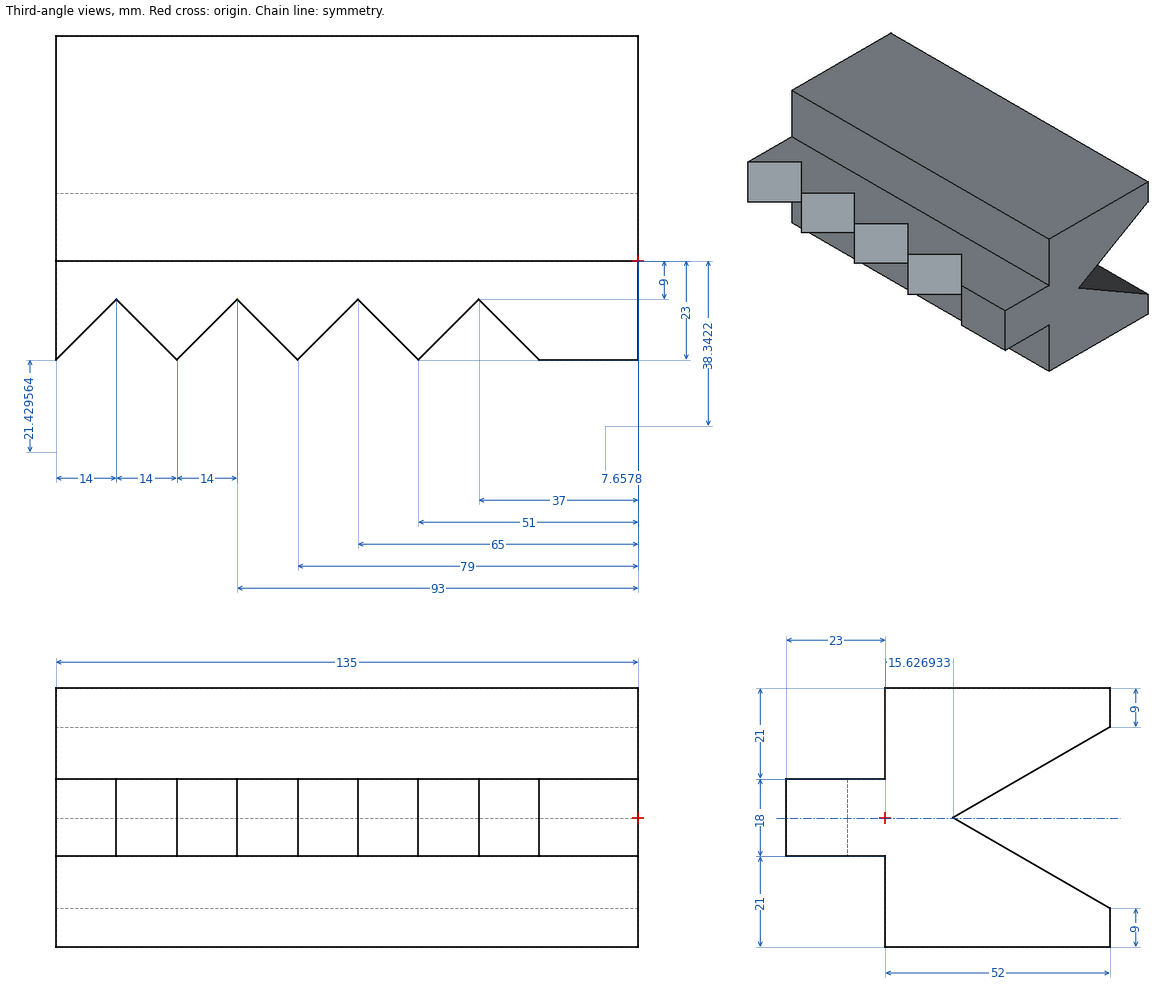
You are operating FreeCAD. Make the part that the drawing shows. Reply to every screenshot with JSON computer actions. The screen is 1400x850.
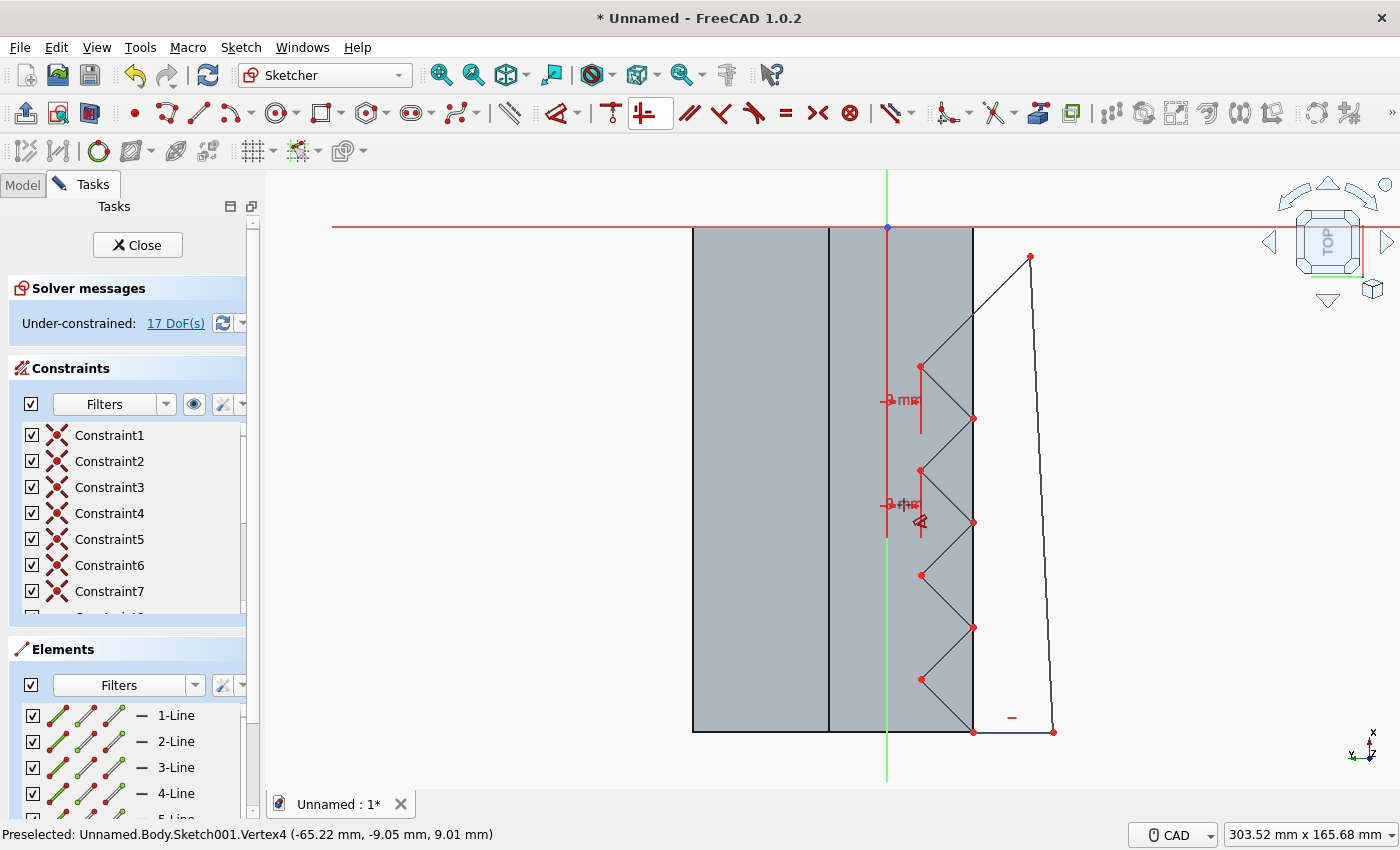
{"action": "left_click", "coordinate": [921, 576]}
{"action": "left_click", "coordinate": [904, 610]}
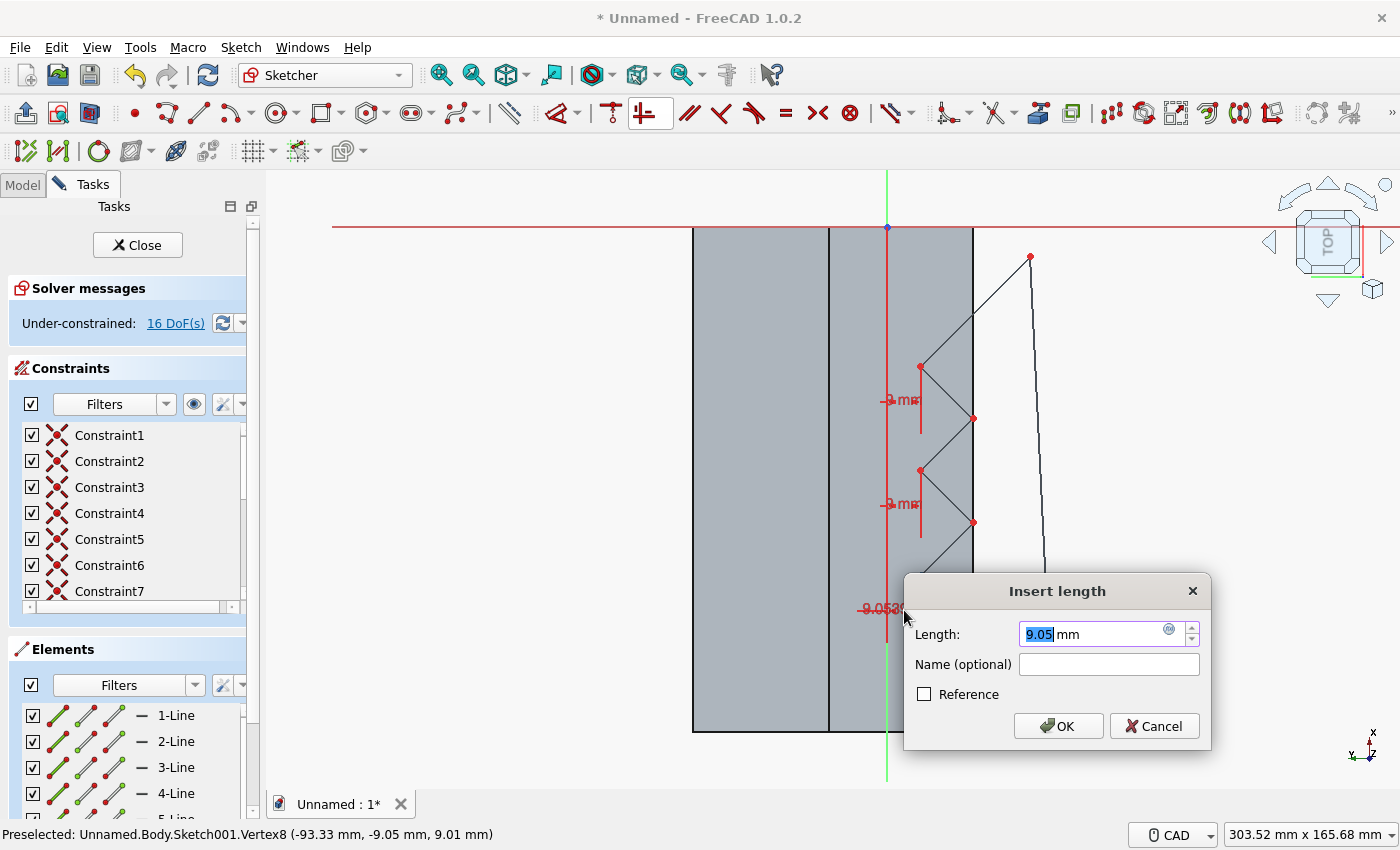
{"action": "type", "text": "9"}
{"action": "key", "text": "Return"}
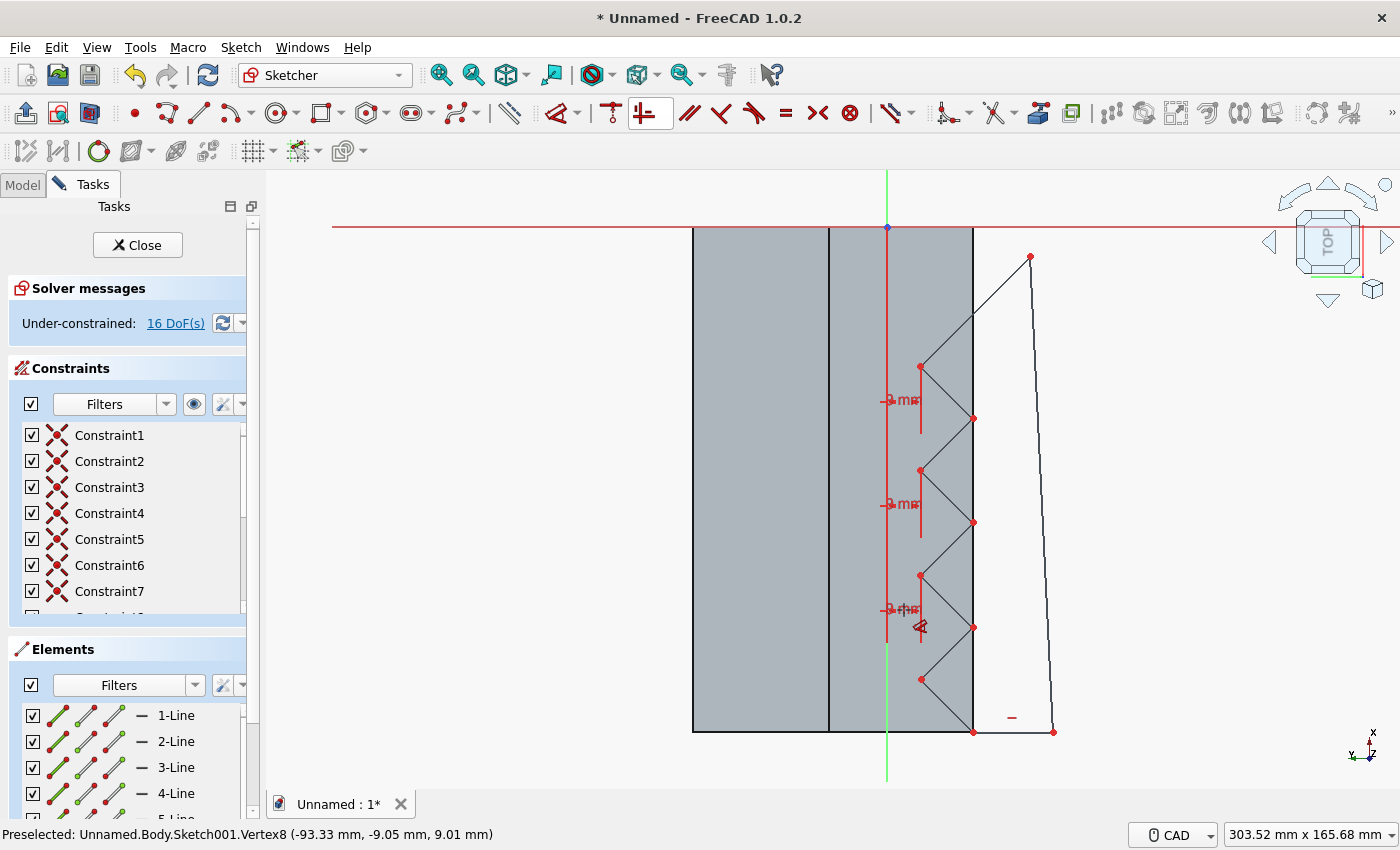
{"action": "left_click", "coordinate": [921, 680]}
{"action": "left_click", "coordinate": [904, 714]}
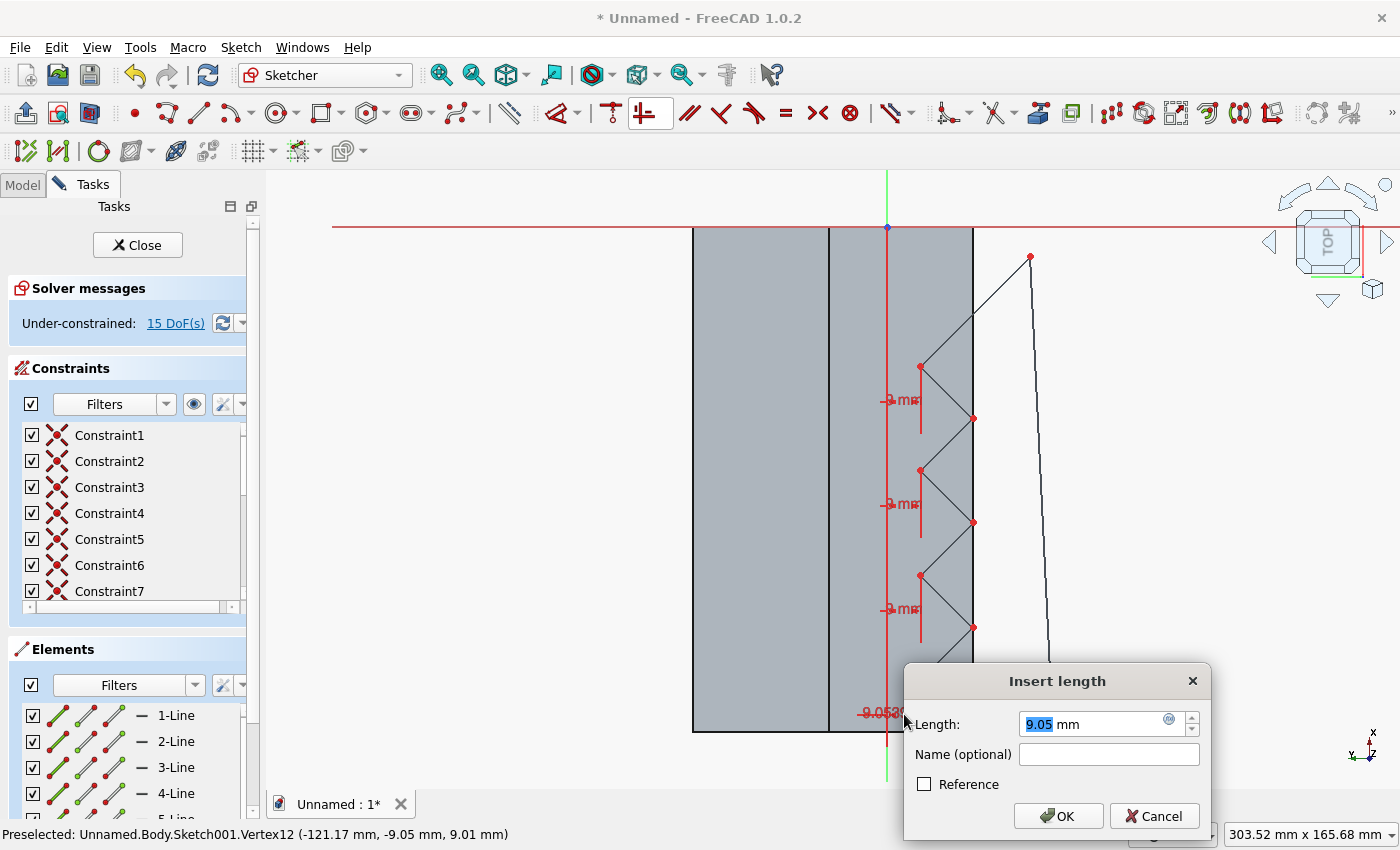
{"action": "type", "text": "9"}
{"action": "key", "text": "Return"}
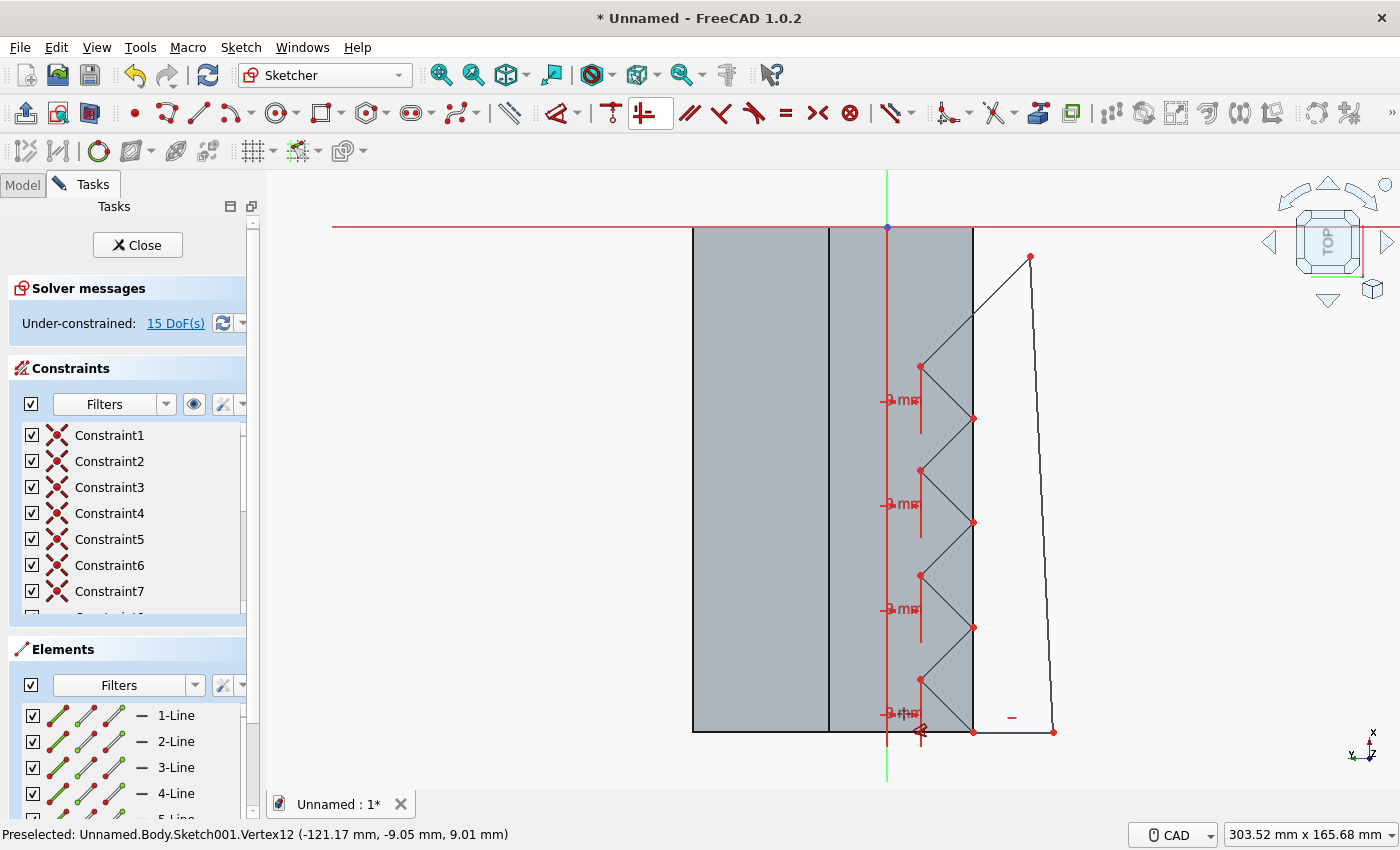
{"action": "left_click", "coordinate": [921, 367]}
{"action": "left_click", "coordinate": [853, 297]}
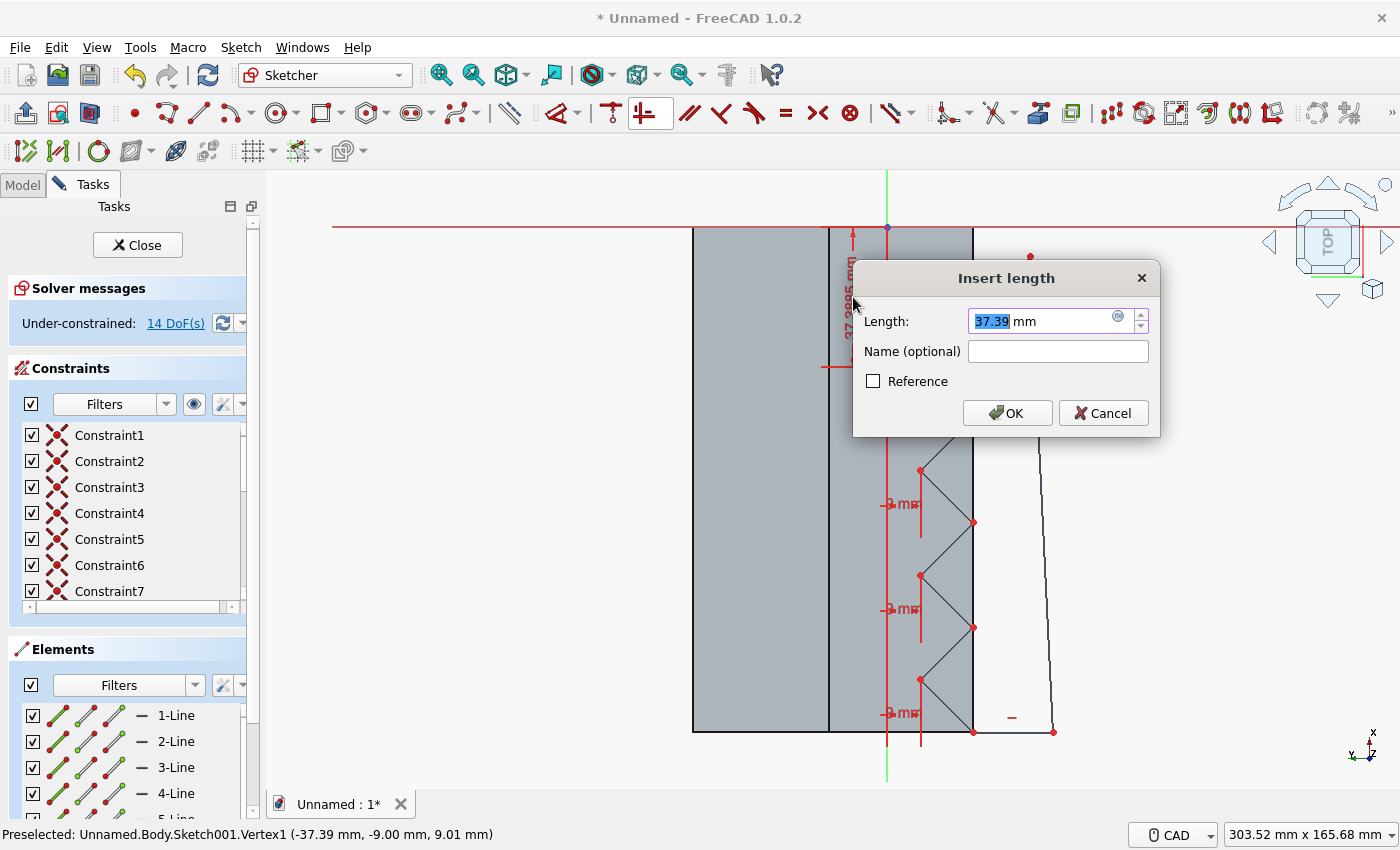
{"action": "type", "text": "37"}
{"action": "key", "text": "Return"}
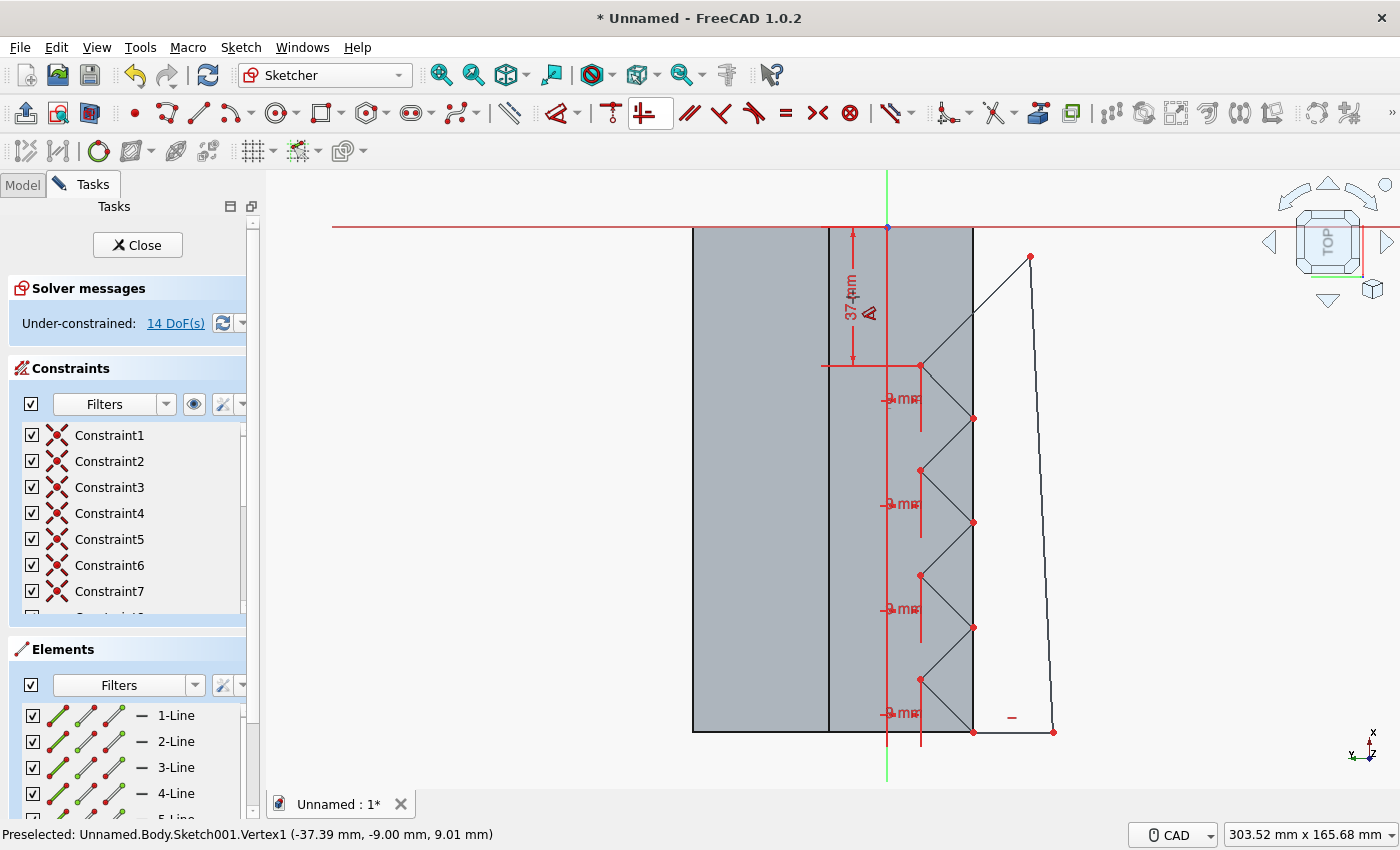
{"action": "left_click", "coordinate": [973, 419]}
{"action": "left_click", "coordinate": [910, 453]}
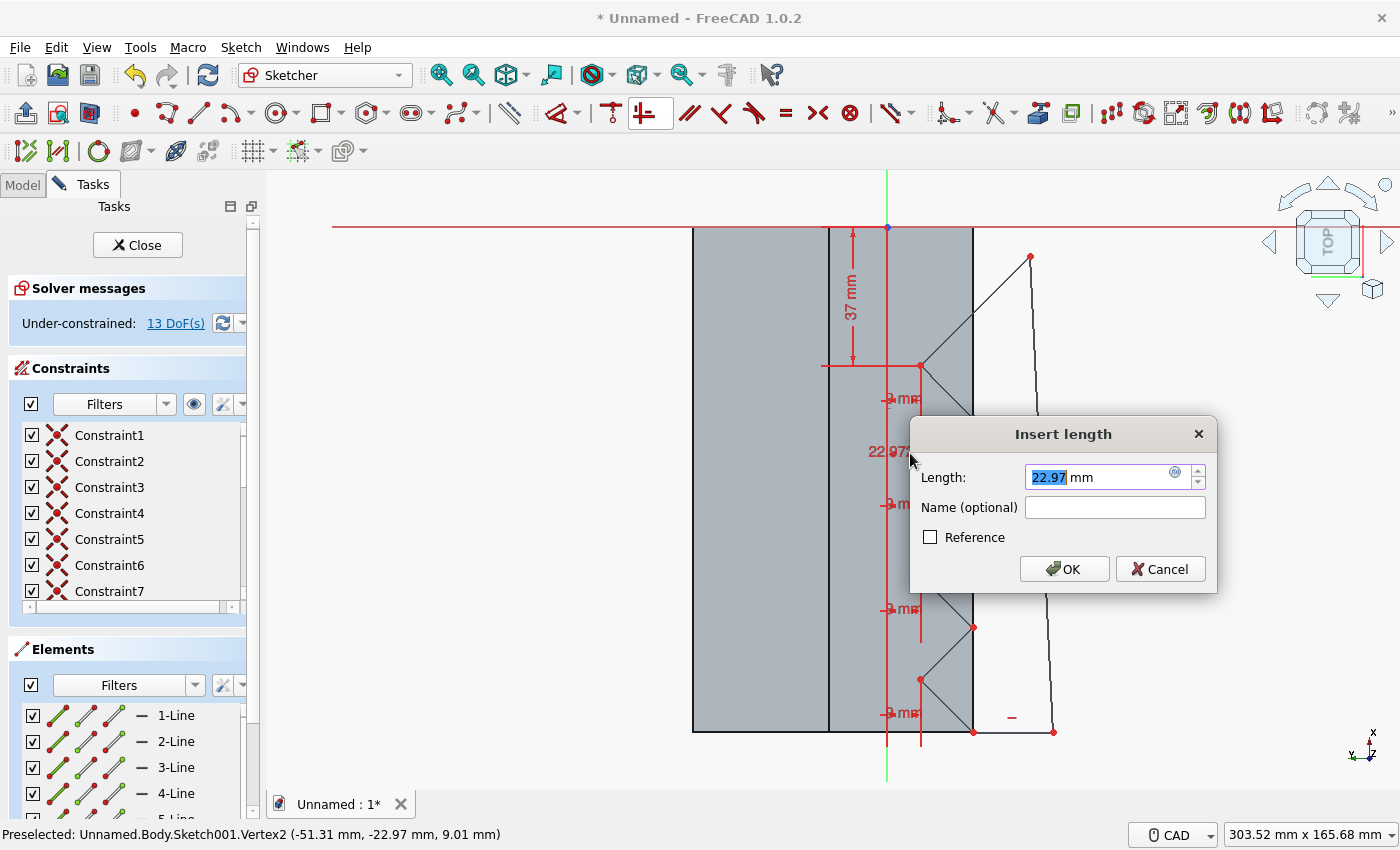
{"action": "type", "text": "23"}
{"action": "key", "text": "Return"}